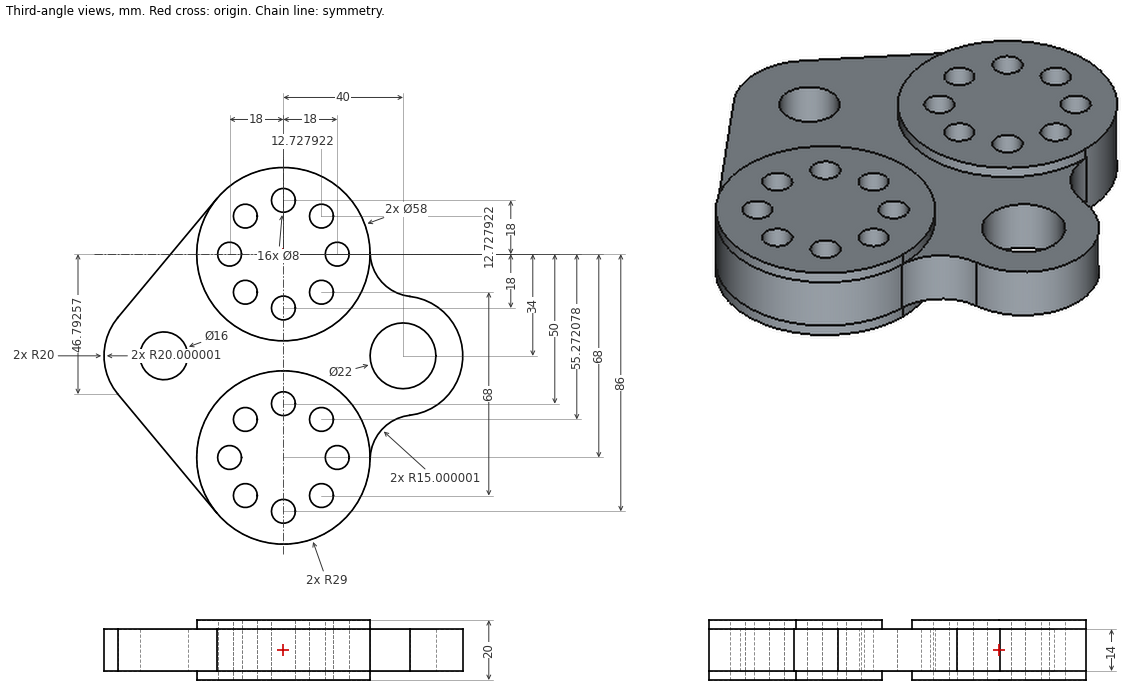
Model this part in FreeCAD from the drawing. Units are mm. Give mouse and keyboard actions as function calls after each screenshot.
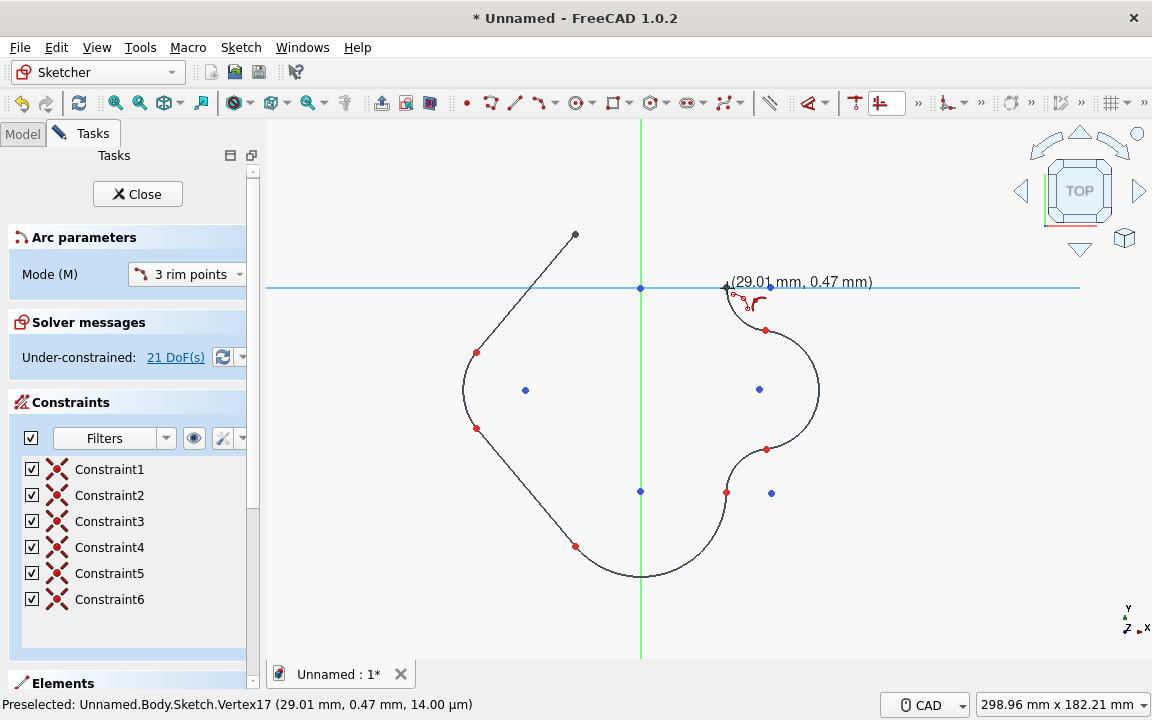
click(575, 234)
click(669, 207)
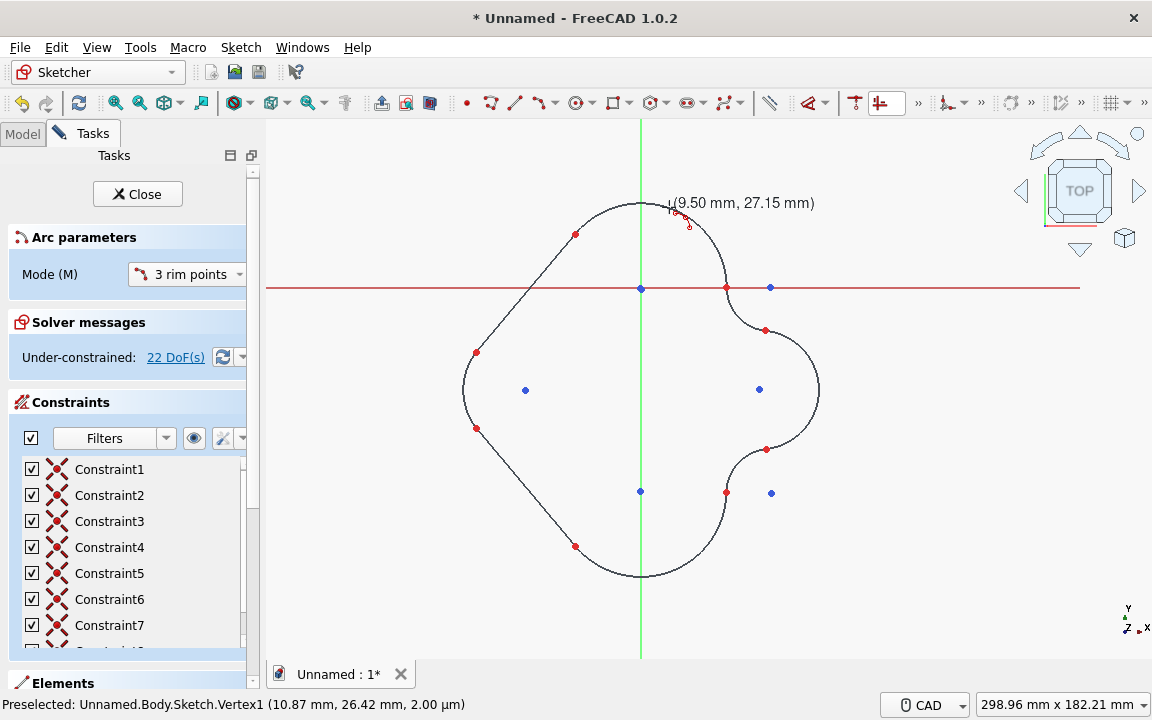
key(g)
key(c)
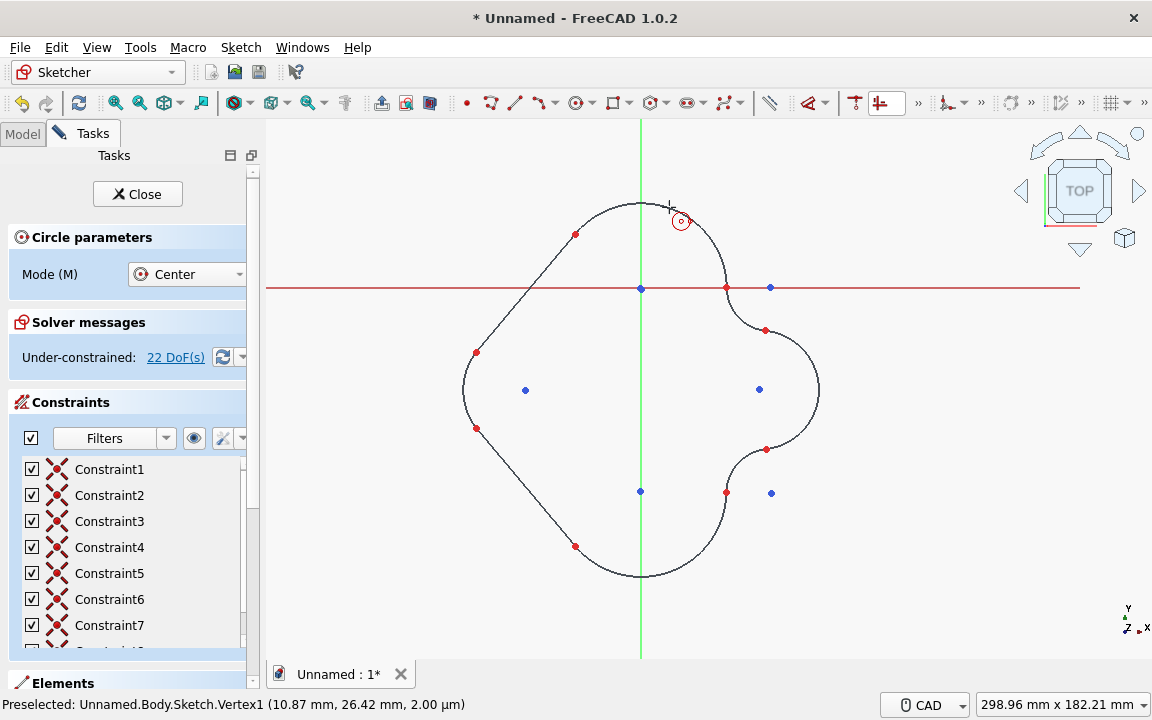
click(759, 389)
move(782, 366)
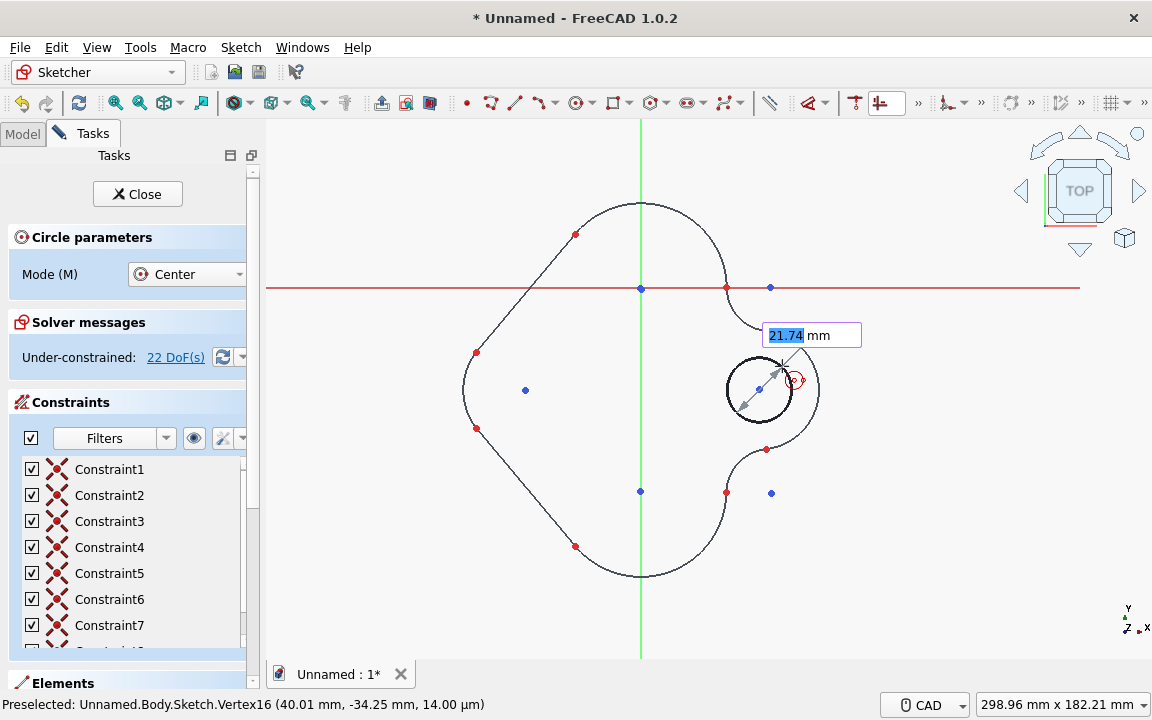
text(22)
key(Return)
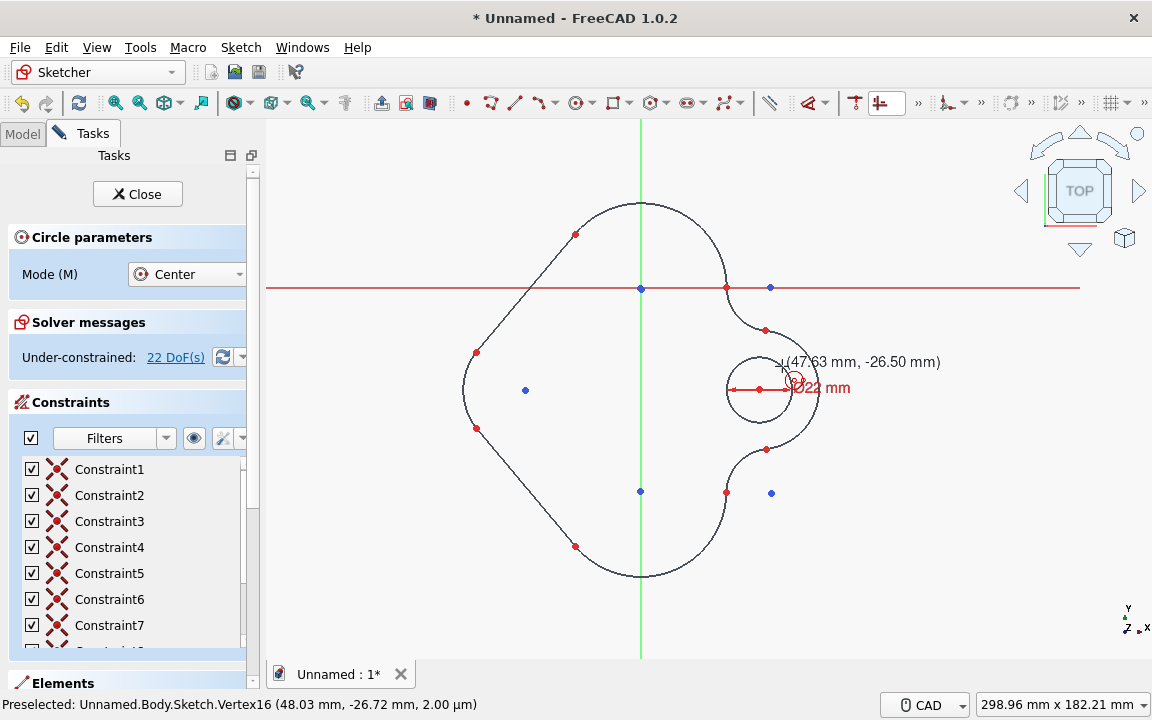
click(522, 389)
move(539, 372)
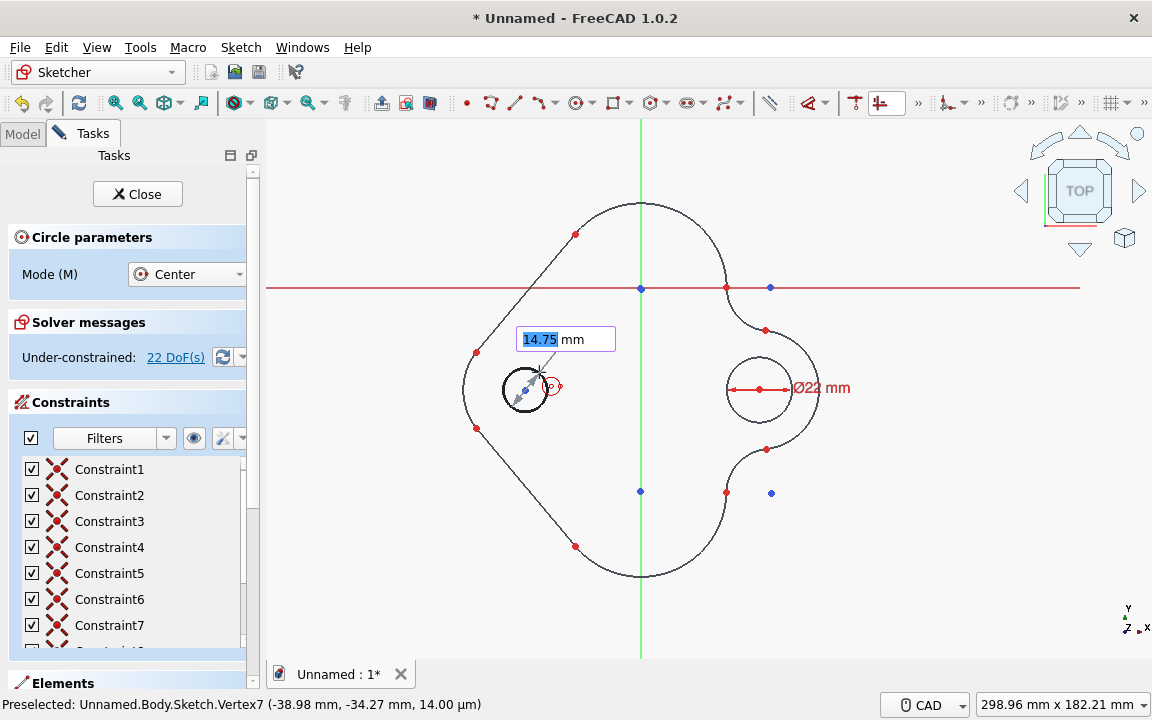
text(16)
key(Return)
key(Escape)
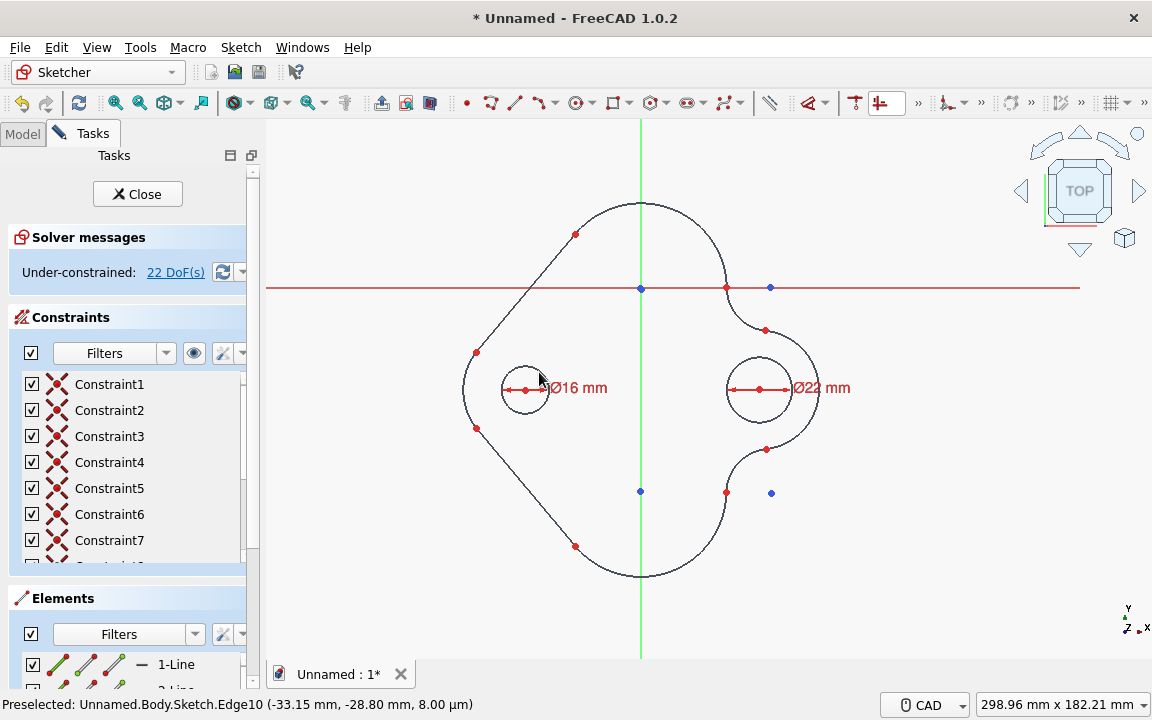
click(546, 269)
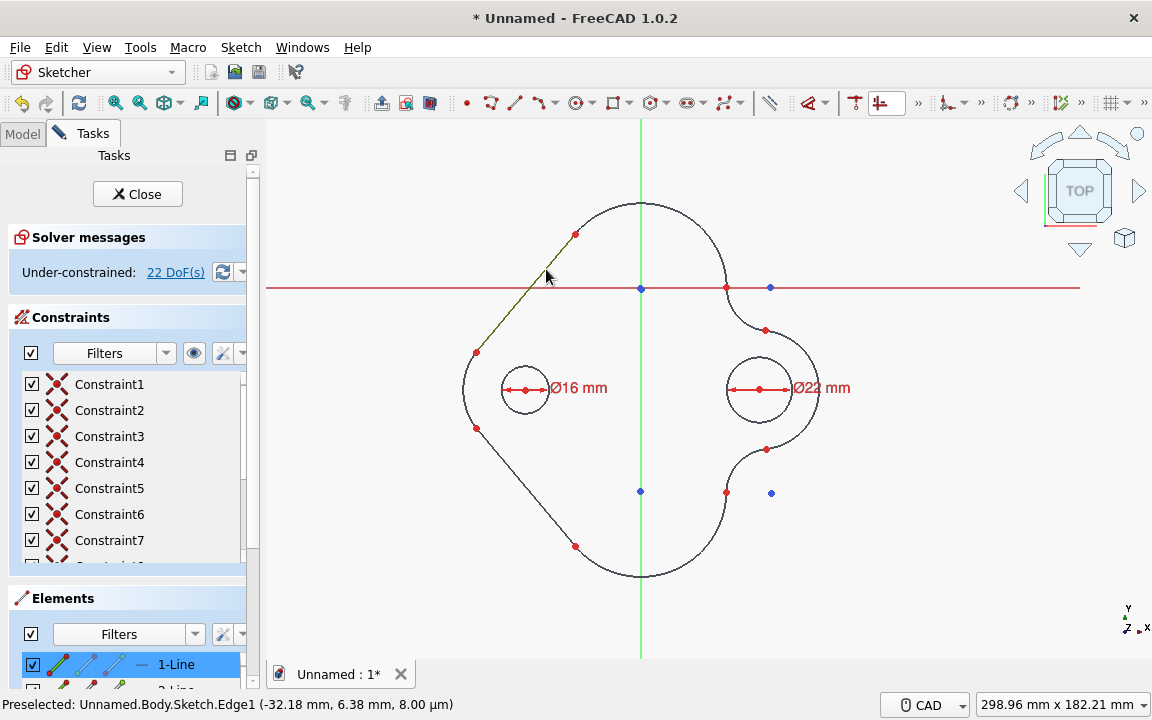
click(465, 374)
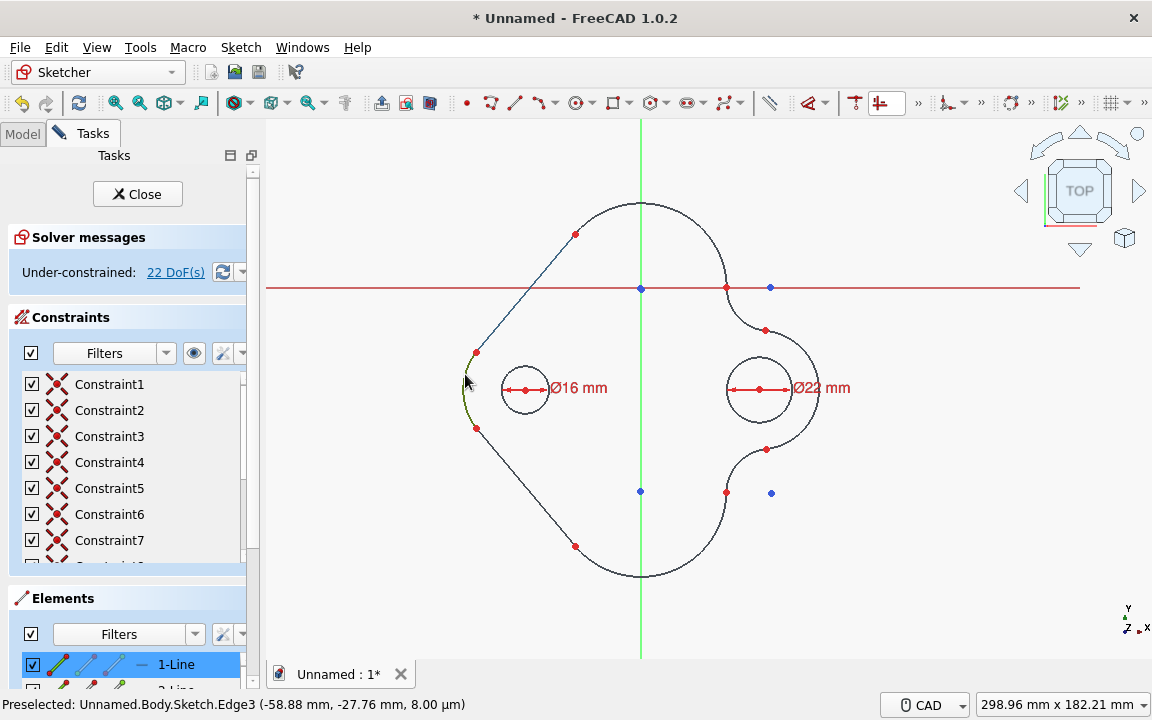
key(t)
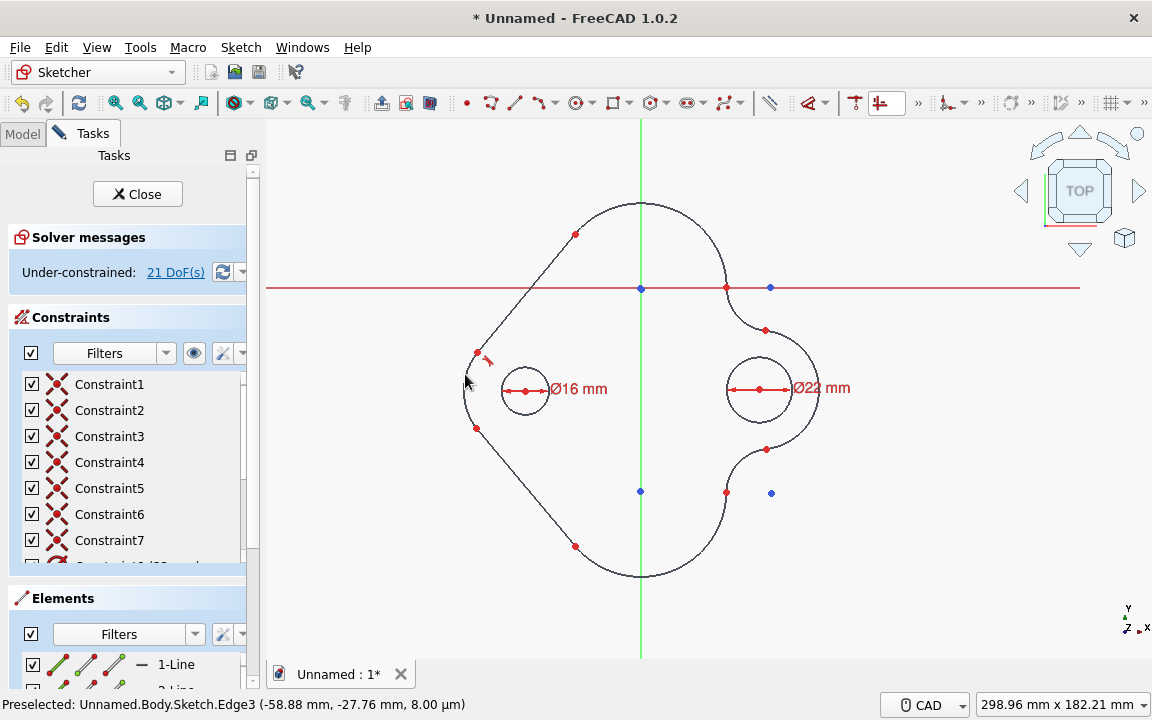
click(546, 269)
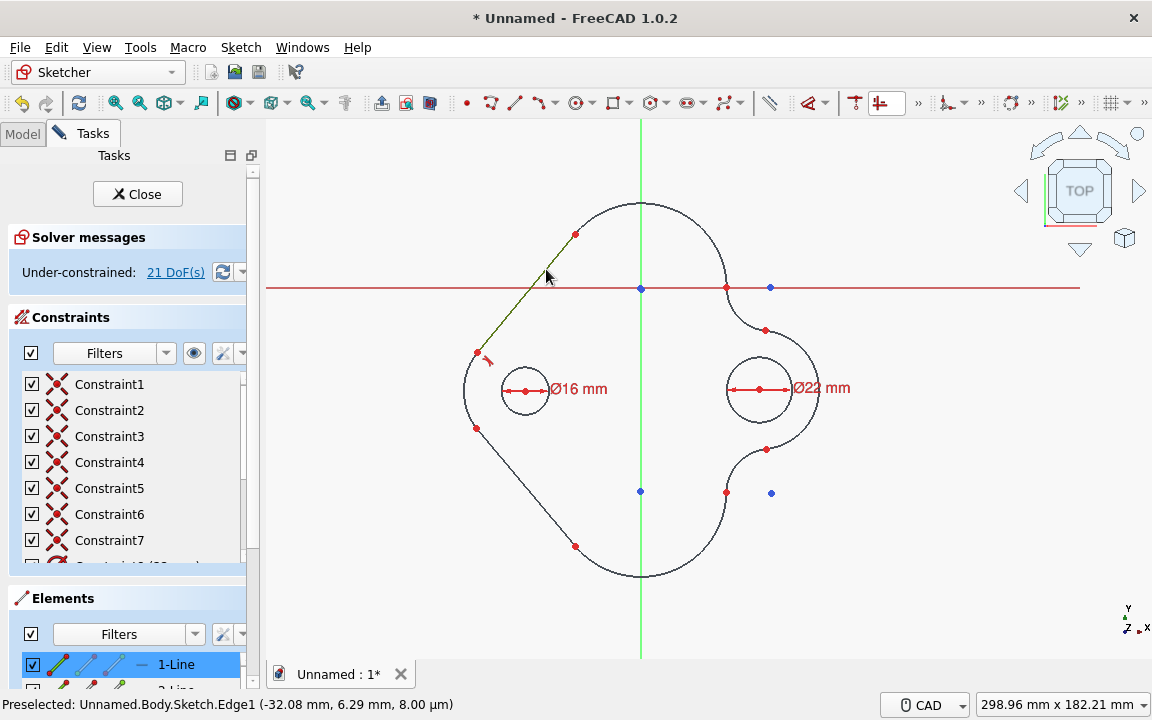
click(704, 231)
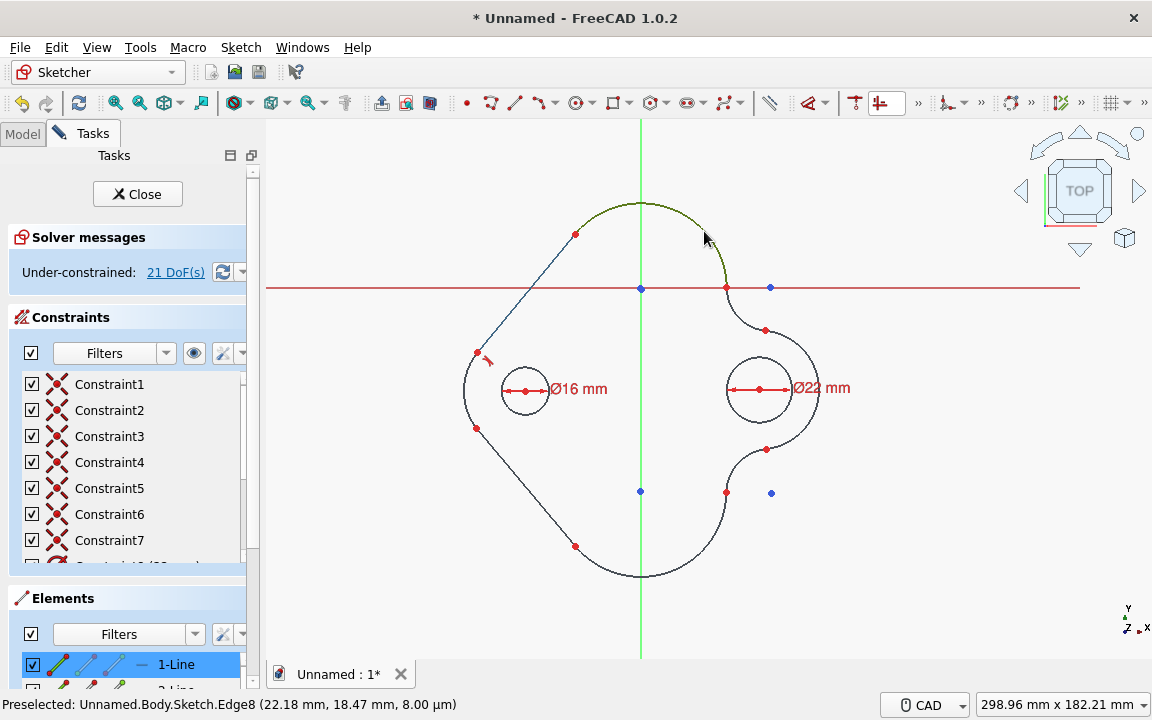
key(t)